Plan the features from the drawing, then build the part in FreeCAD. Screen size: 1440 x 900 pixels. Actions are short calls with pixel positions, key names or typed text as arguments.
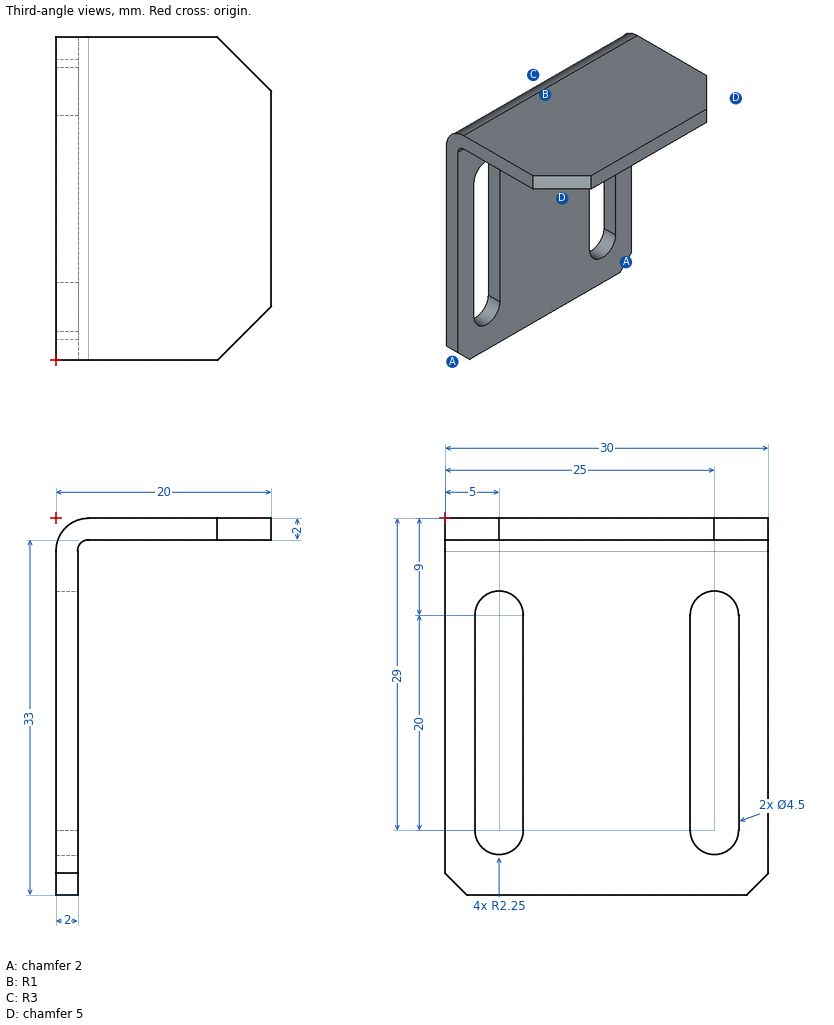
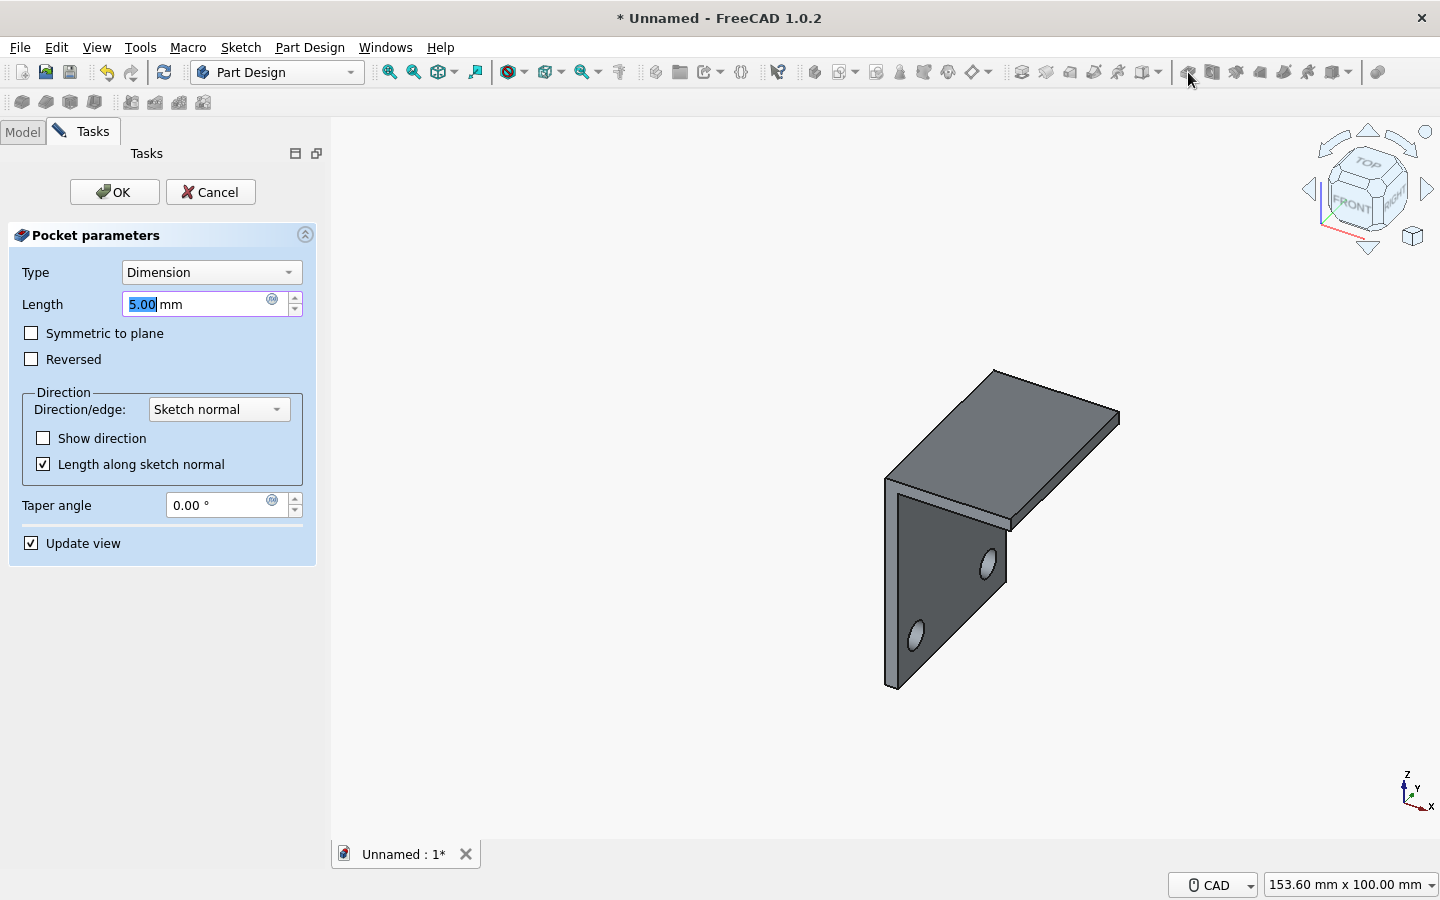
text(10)
key(Tab)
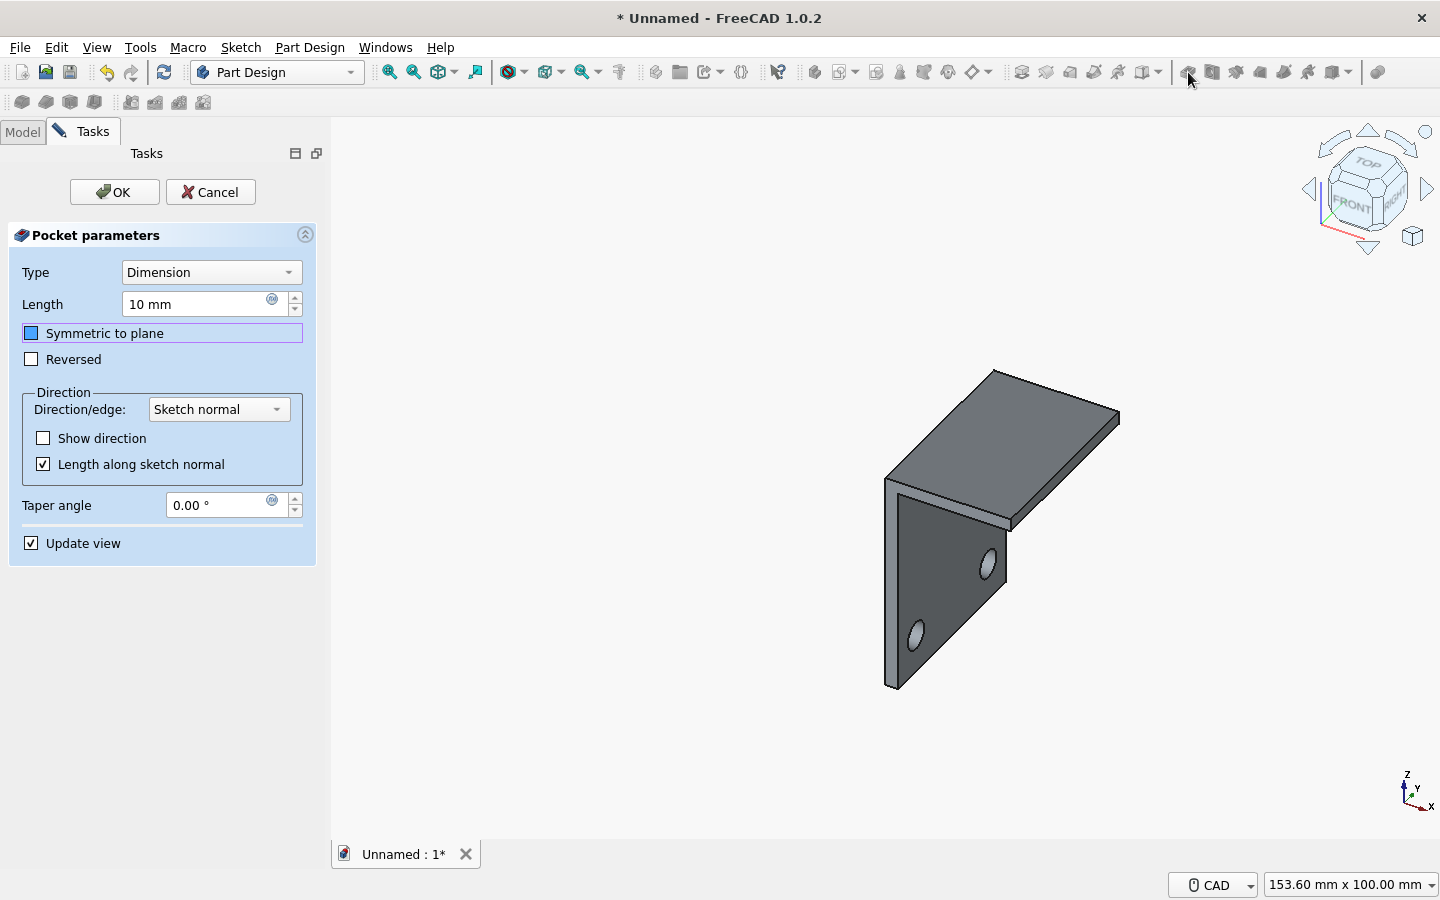
click(115, 192)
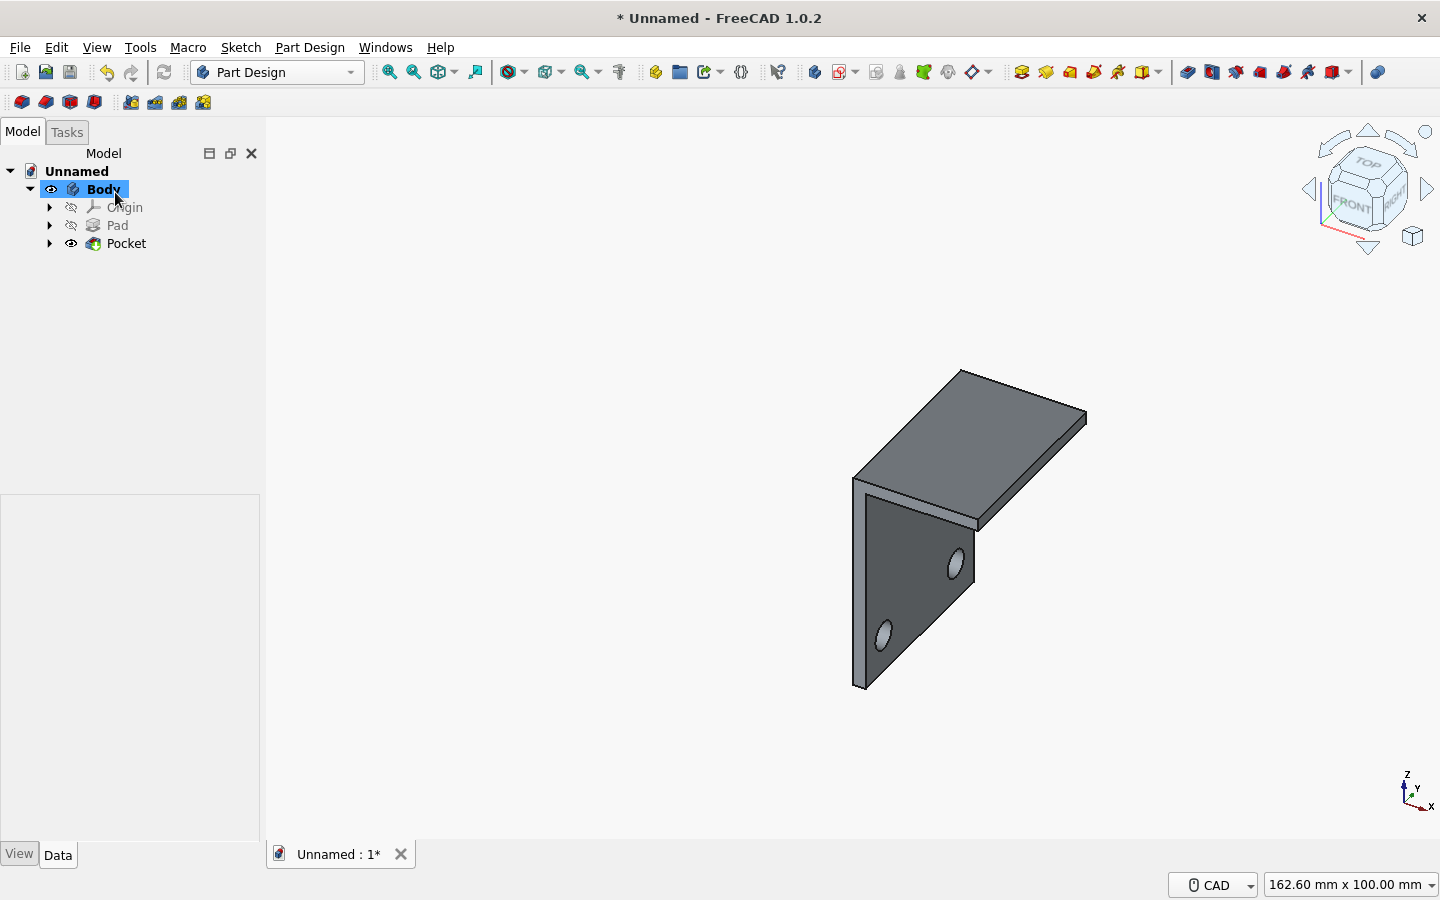
scroll(968, 578, up, 6)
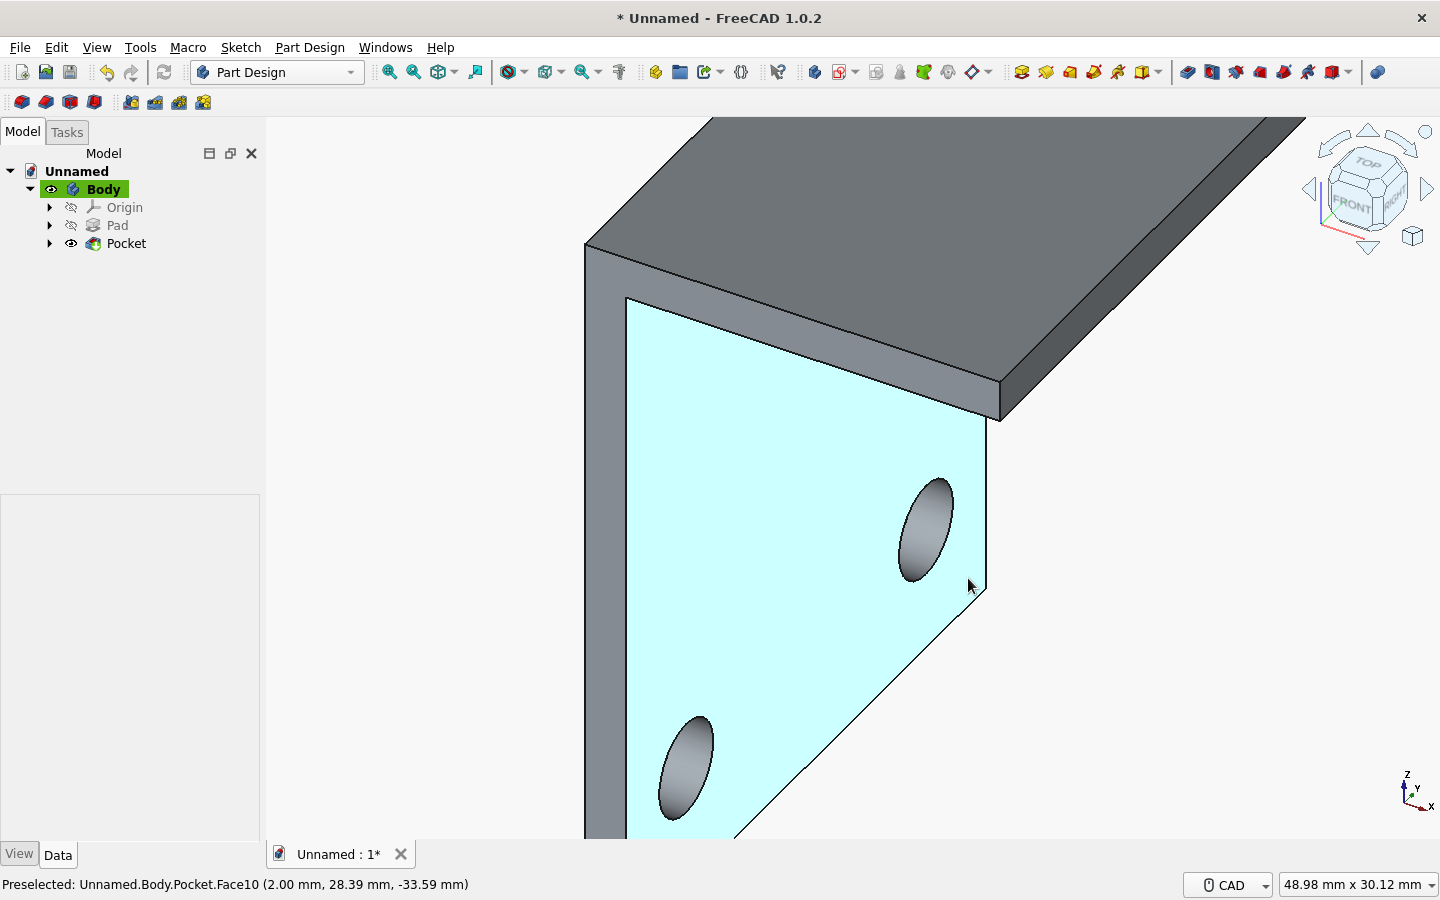
click(390, 72)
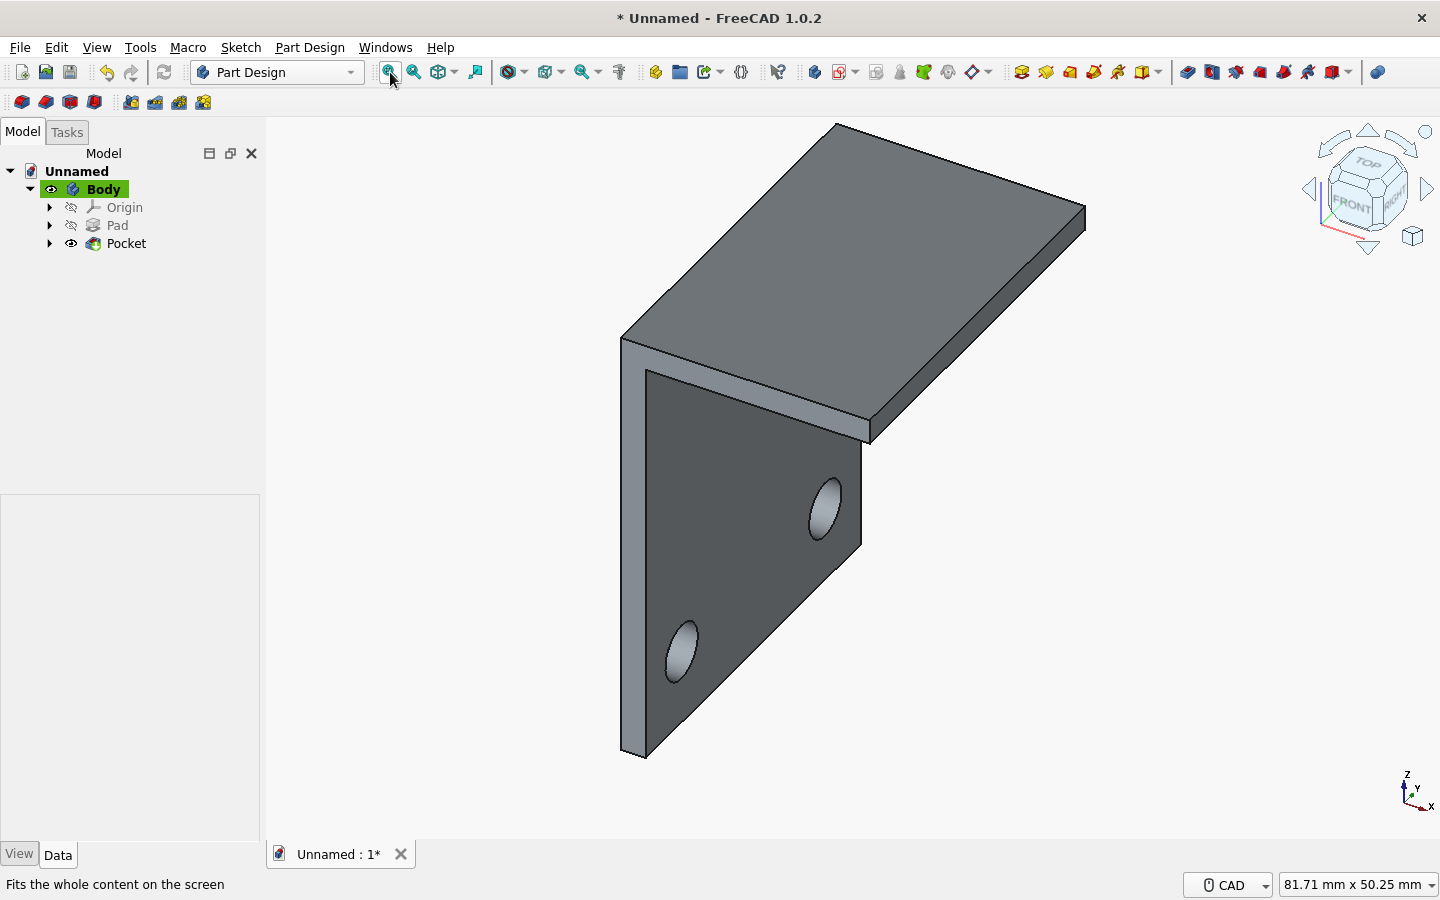
key(0)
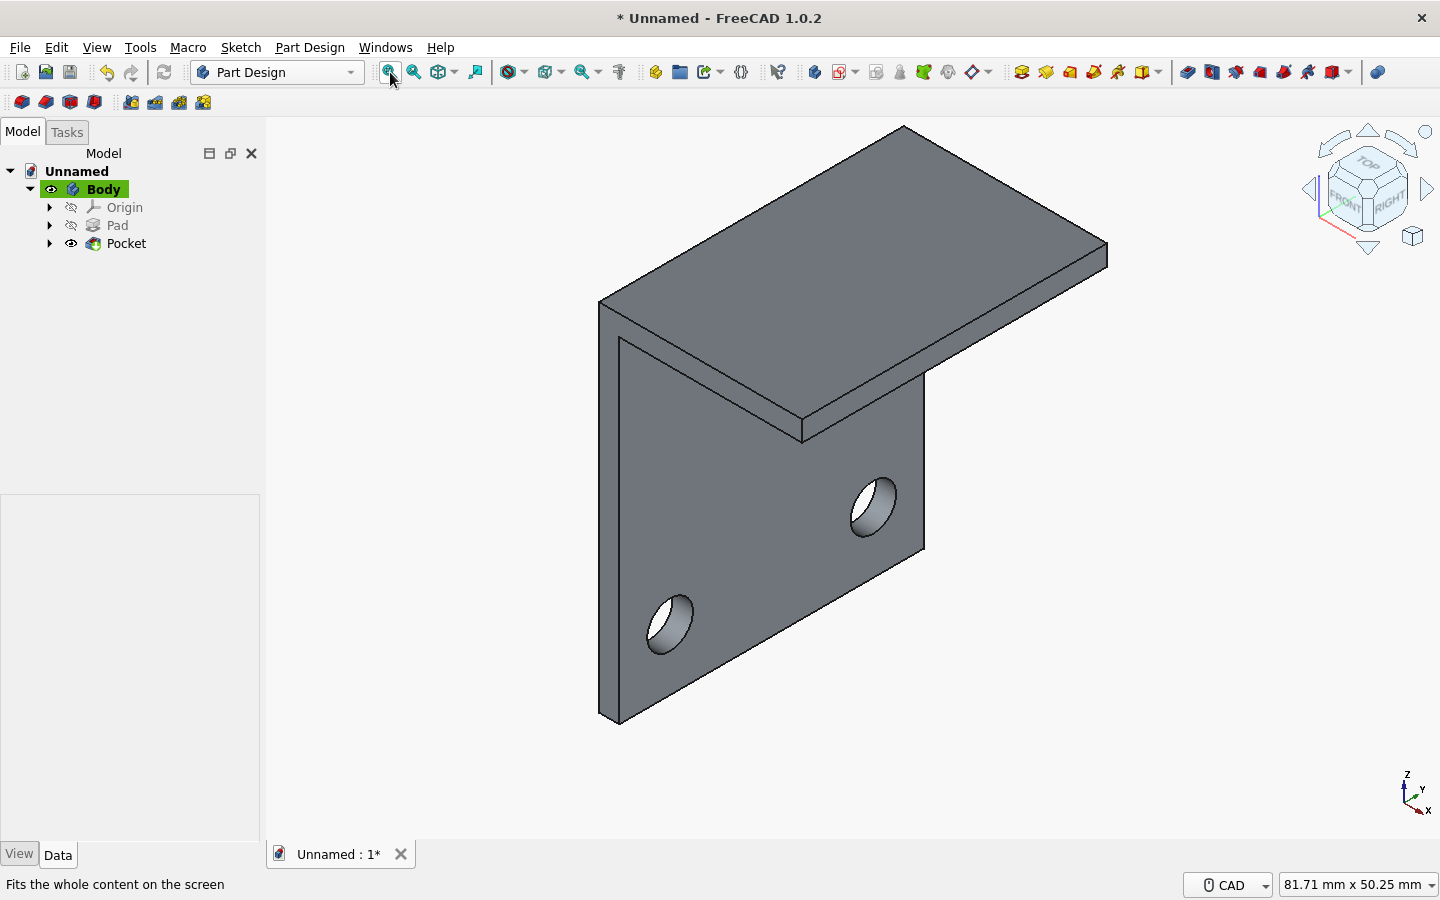
key(2)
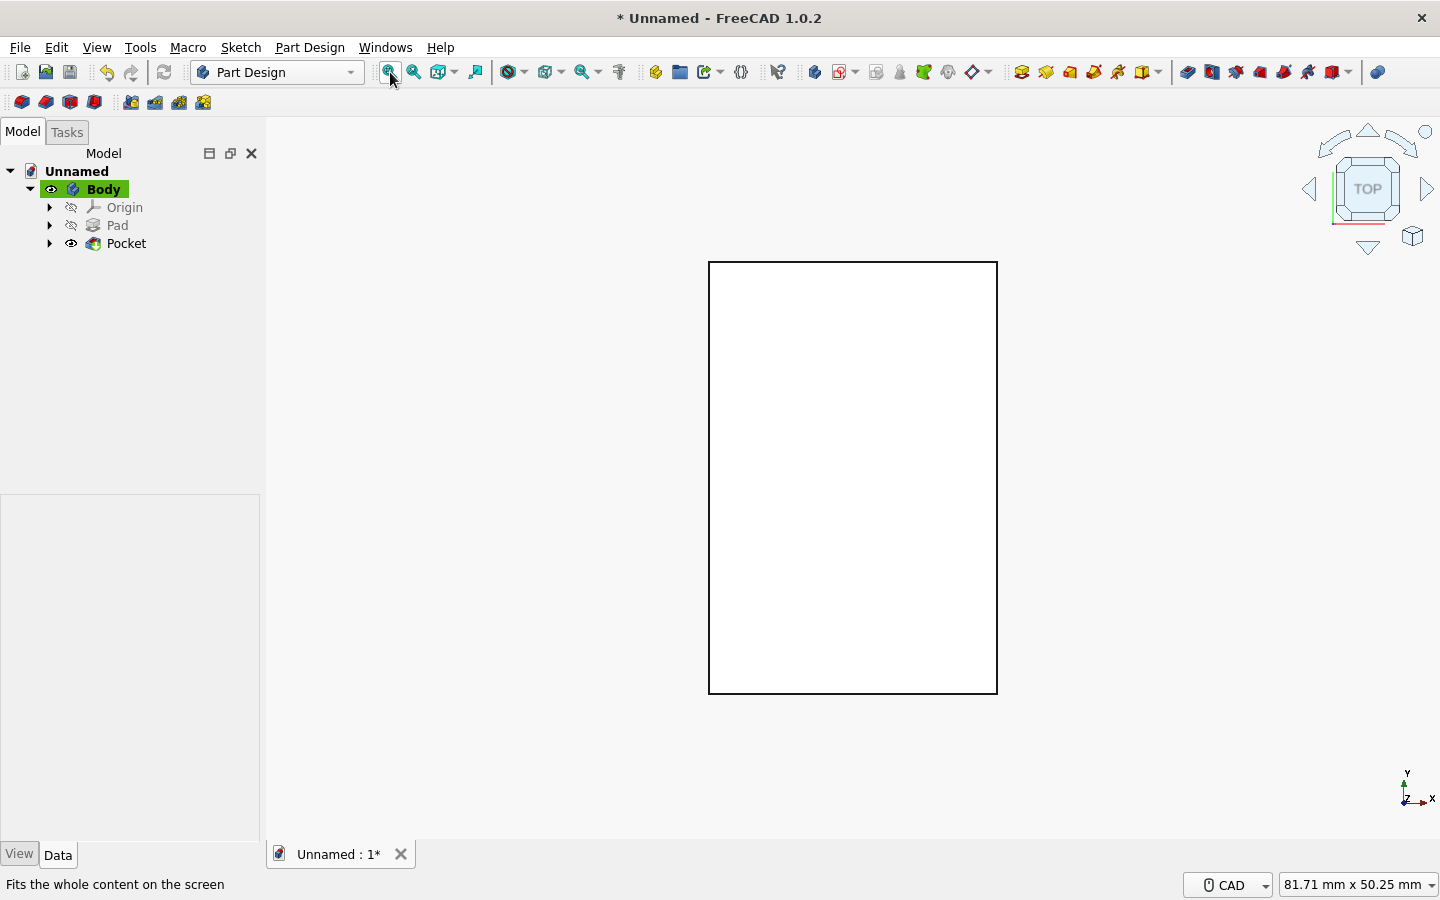
key(1)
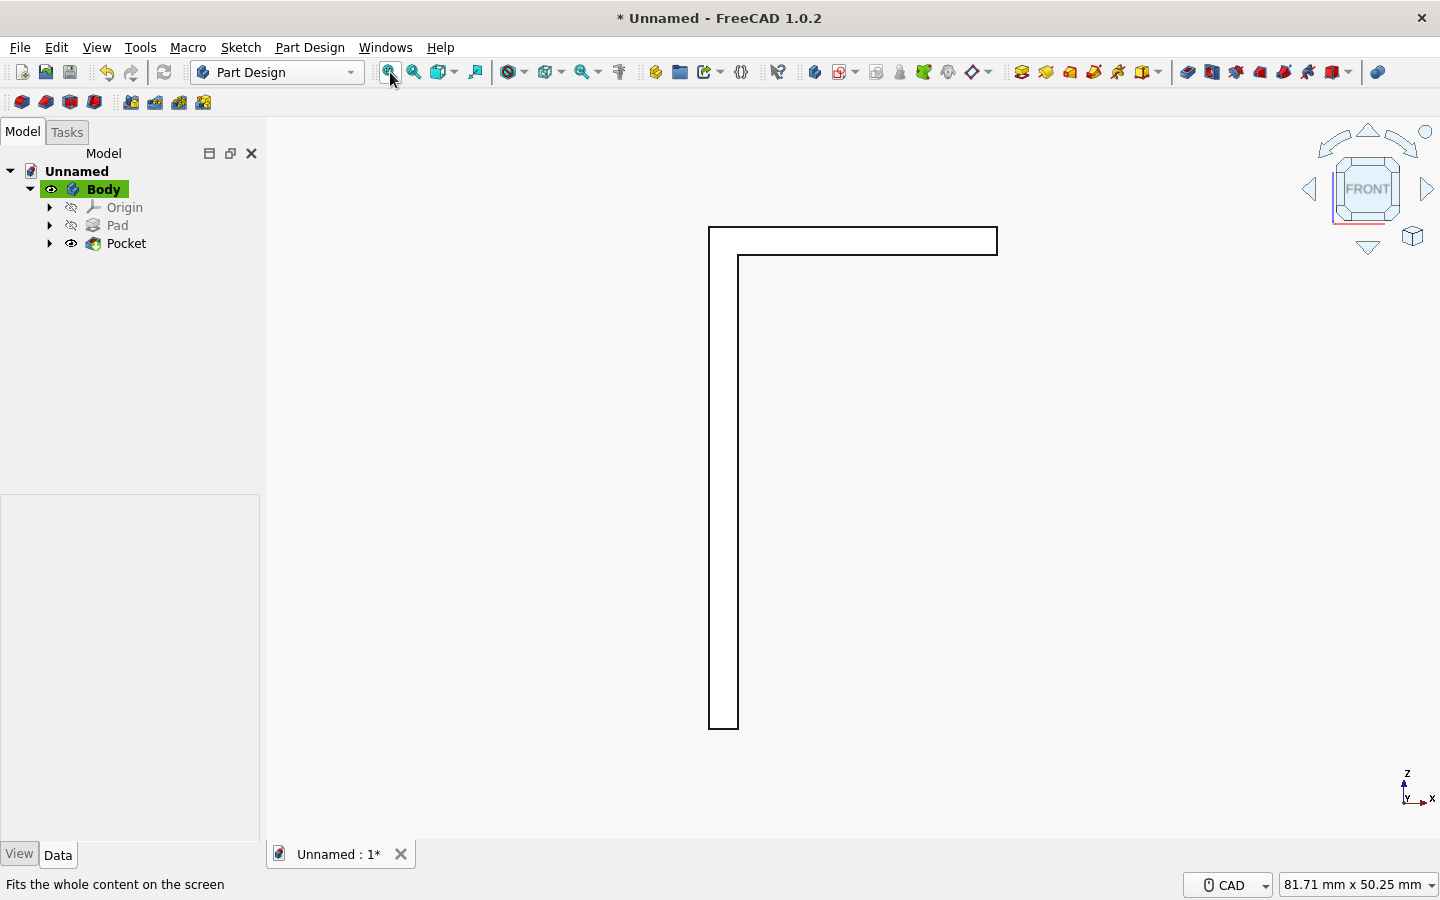
key(3)